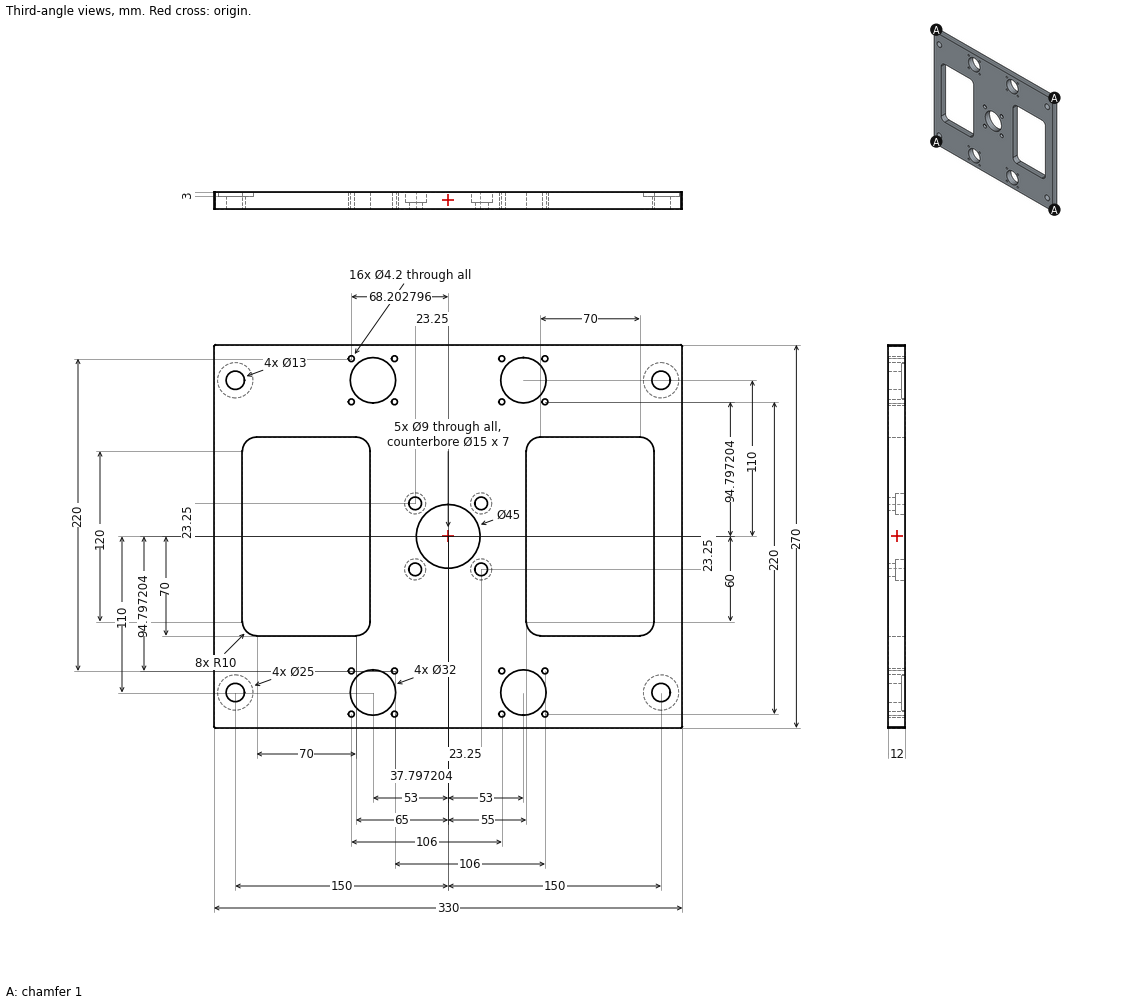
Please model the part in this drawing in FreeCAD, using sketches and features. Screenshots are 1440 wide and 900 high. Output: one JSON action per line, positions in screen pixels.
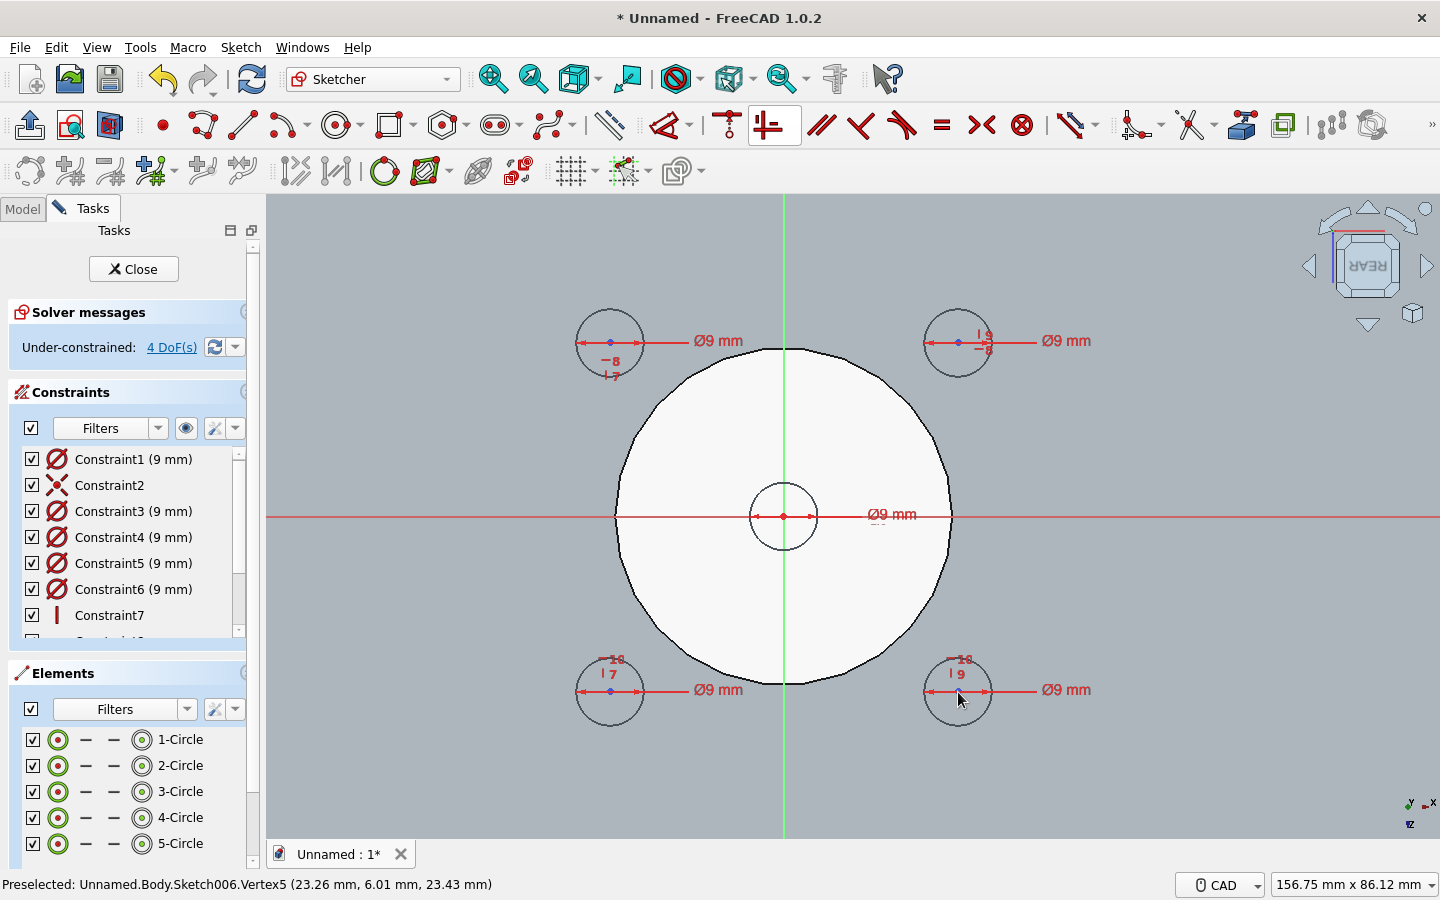
{"action": "left_click", "coordinate": [664, 126]}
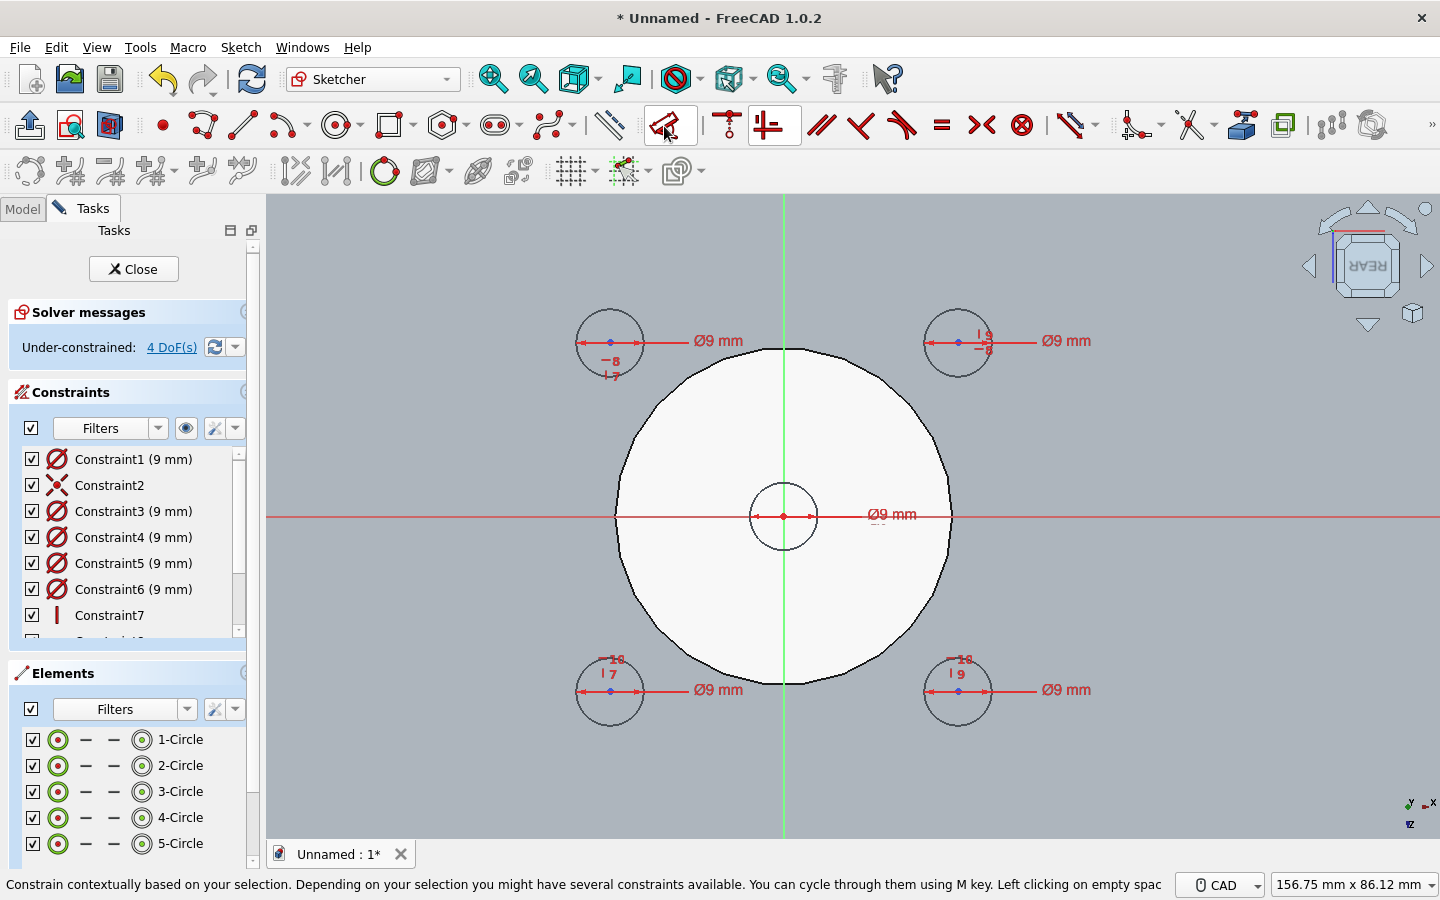
{"action": "left_click", "coordinate": [958, 343]}
{"action": "left_click", "coordinate": [871, 309]}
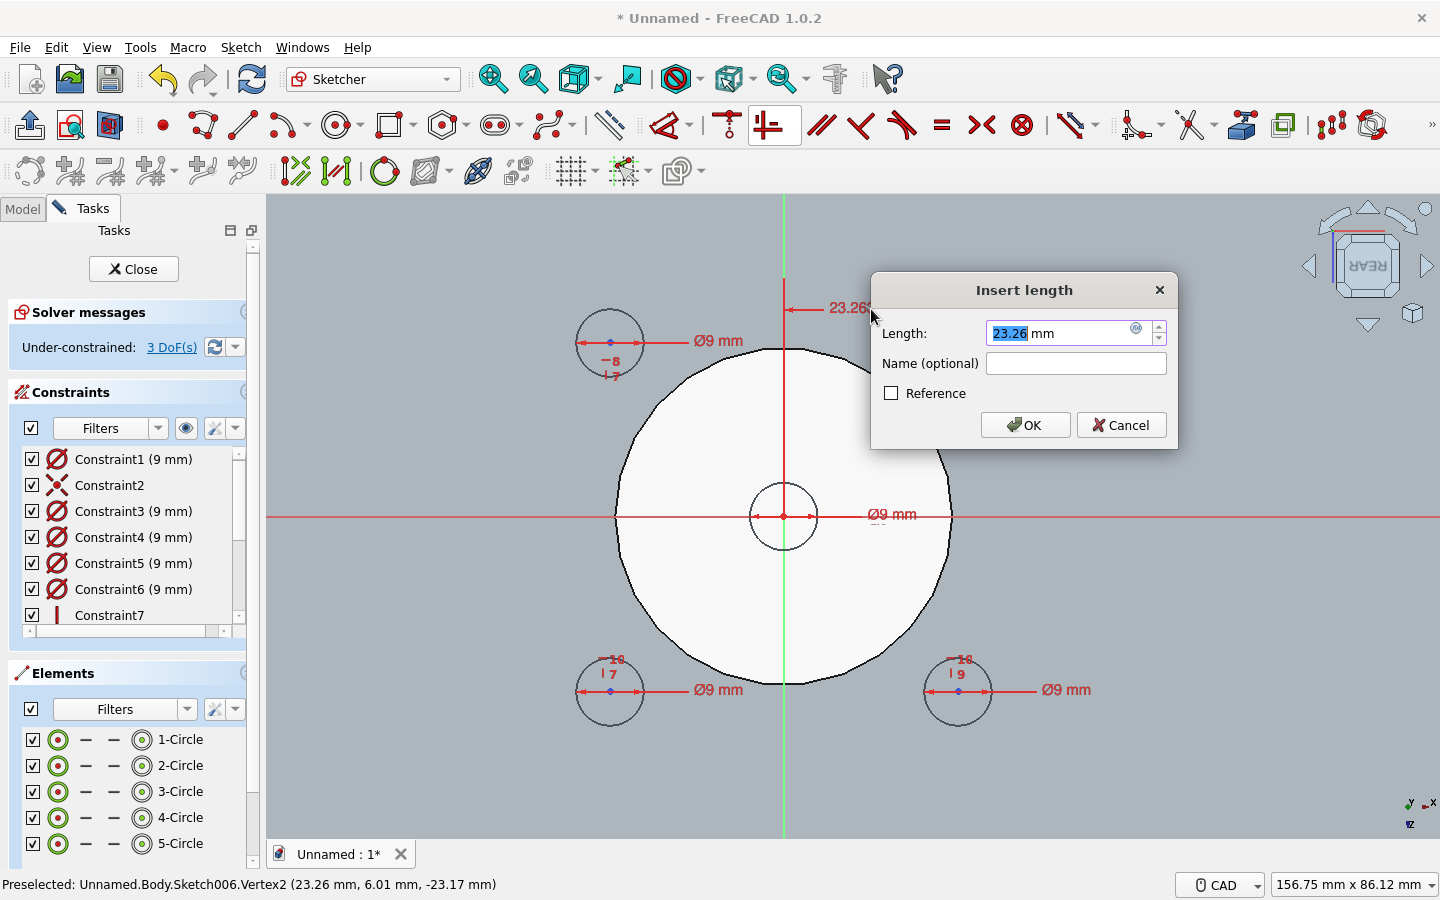
{"action": "type", "text": "23.25"}
{"action": "key", "text": "Return"}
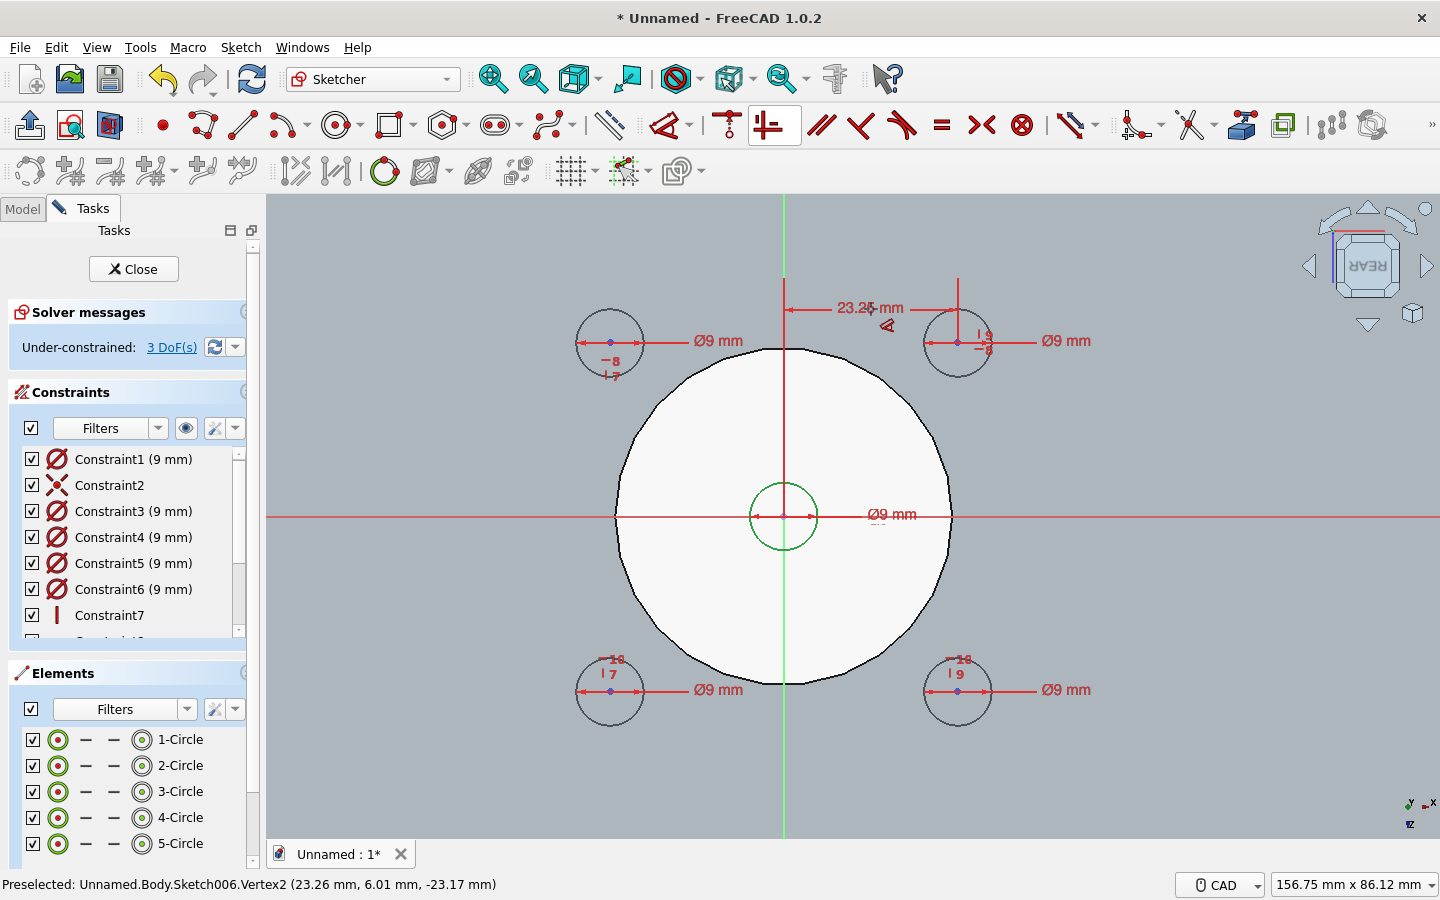
{"action": "left_click", "coordinate": [958, 343]}
{"action": "left_click", "coordinate": [992, 430]}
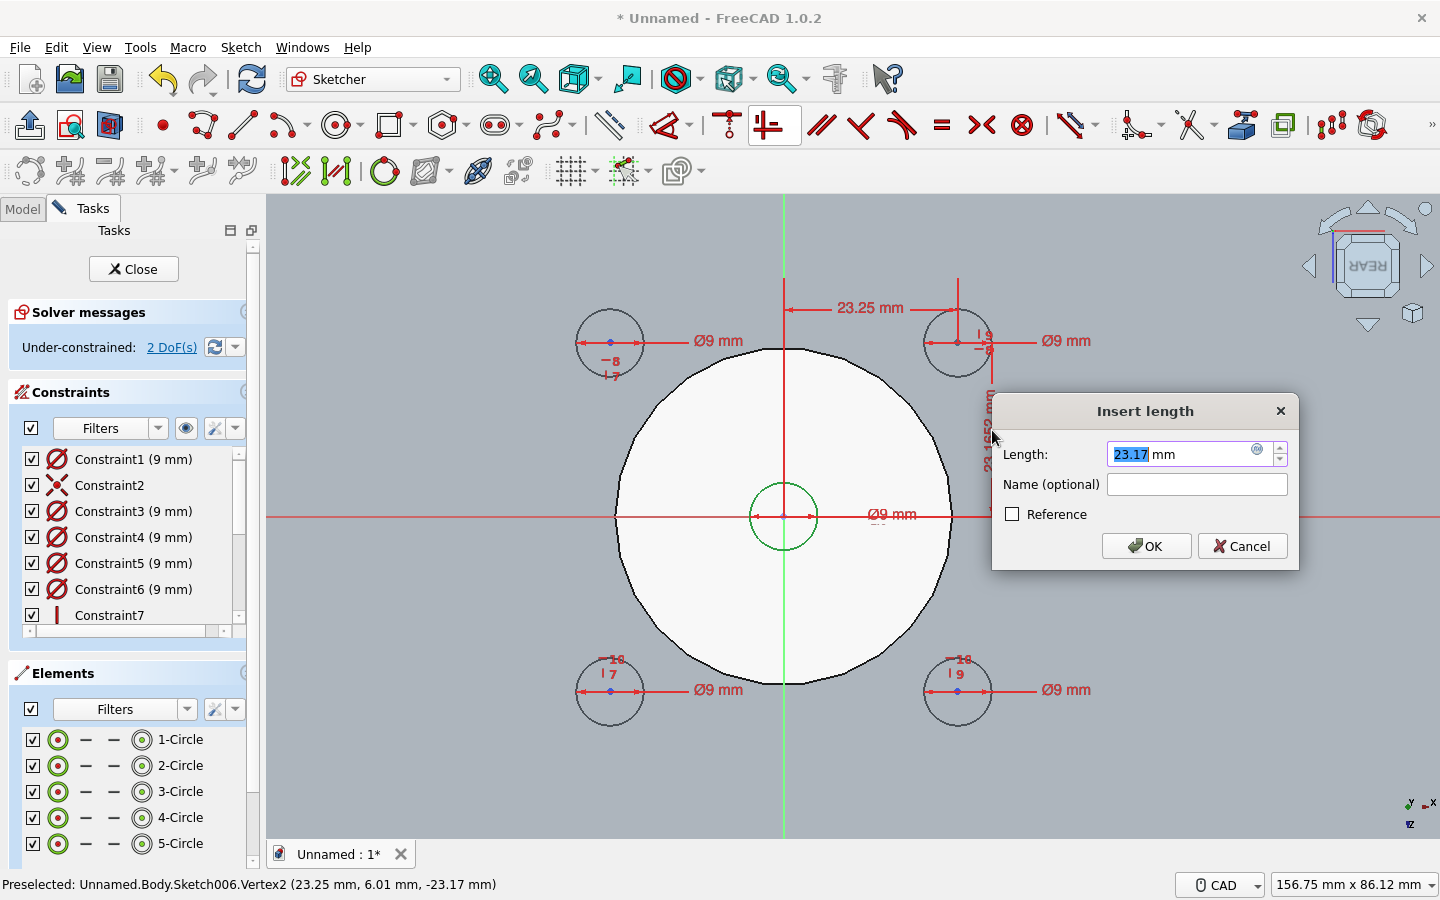
{"action": "type", "text": "23.25"}
{"action": "key", "text": "Return"}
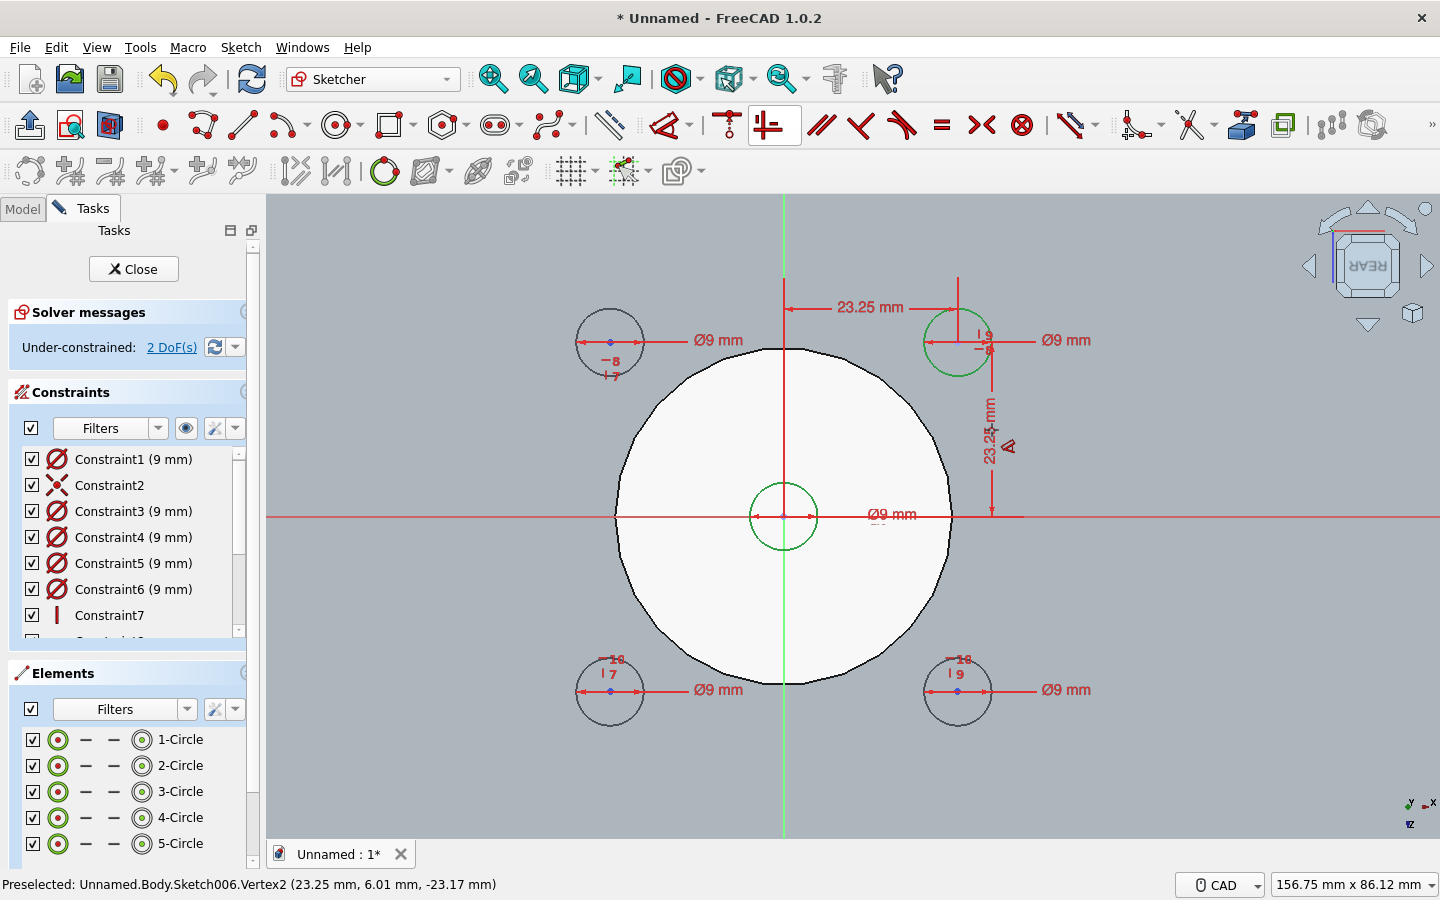
{"action": "left_click", "coordinate": [610, 692]}
{"action": "left_click", "coordinate": [697, 726]}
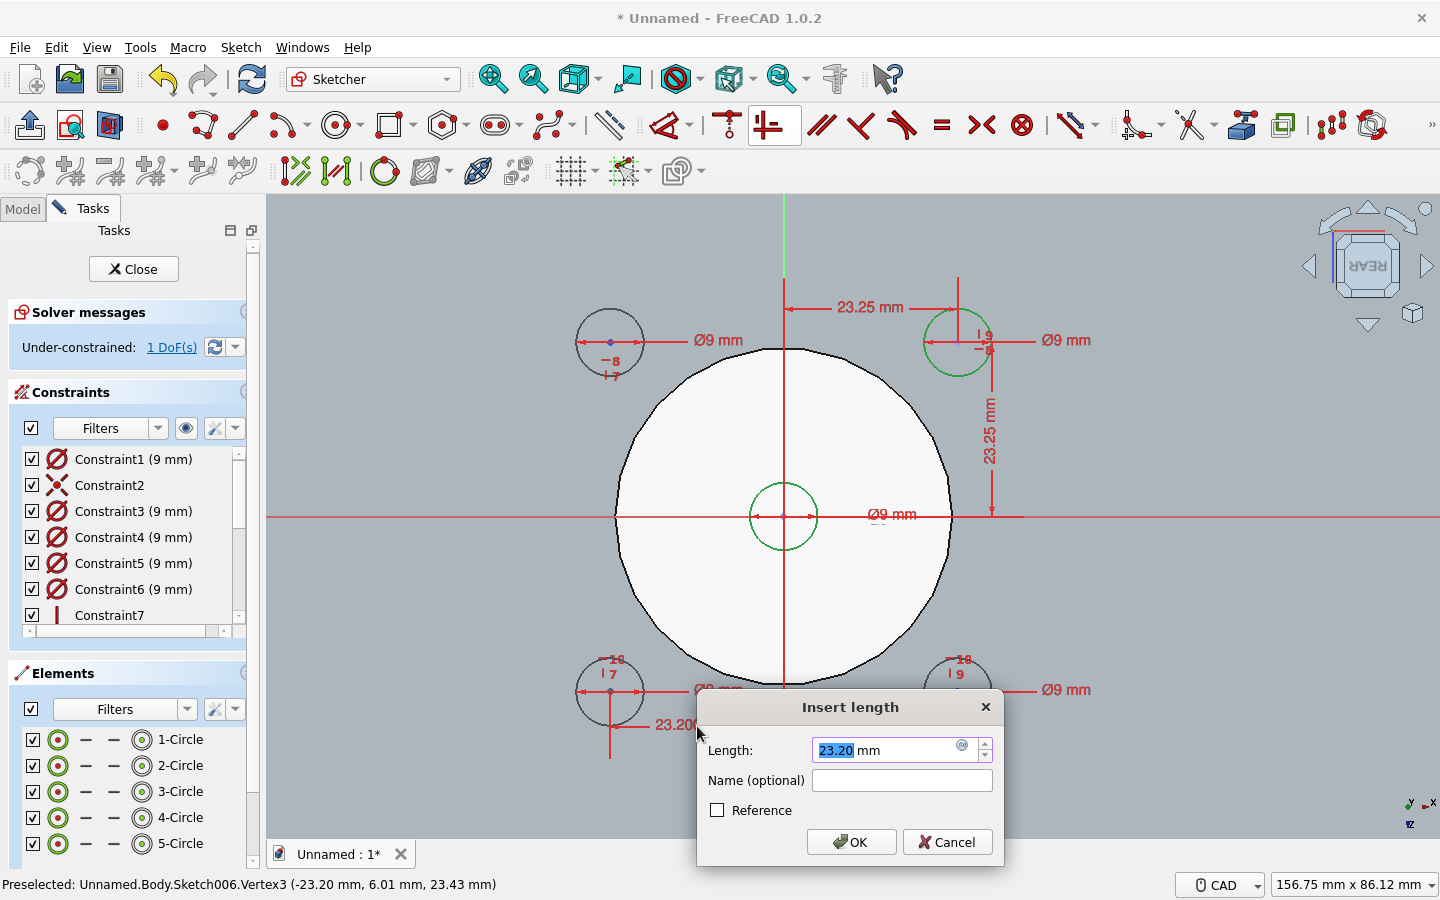
{"action": "type", "text": "23.25"}
{"action": "key", "text": "Return"}